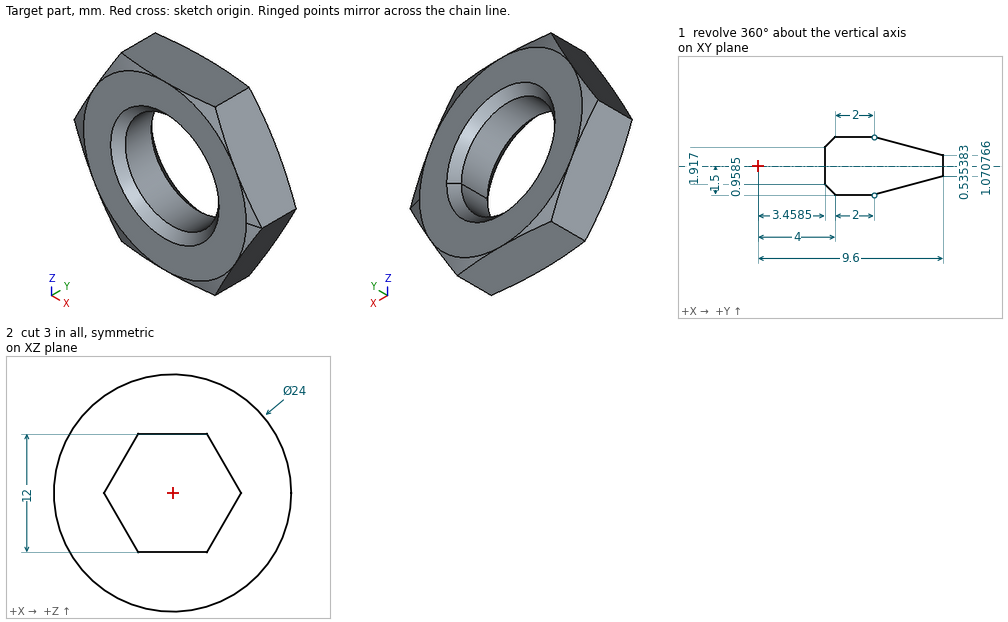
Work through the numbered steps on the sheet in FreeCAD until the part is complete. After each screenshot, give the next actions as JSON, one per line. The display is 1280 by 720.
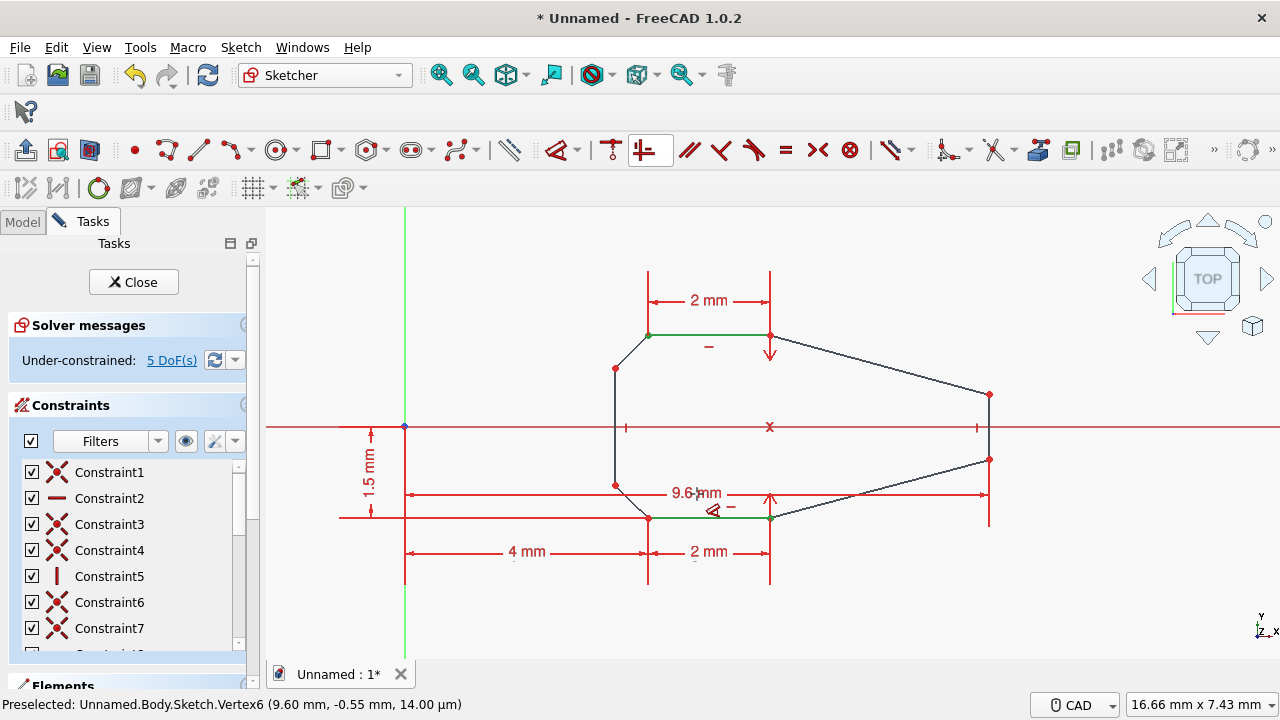
{"action": "left_click", "coordinate": [615, 404]}
{"action": "left_click", "coordinate": [581, 401]}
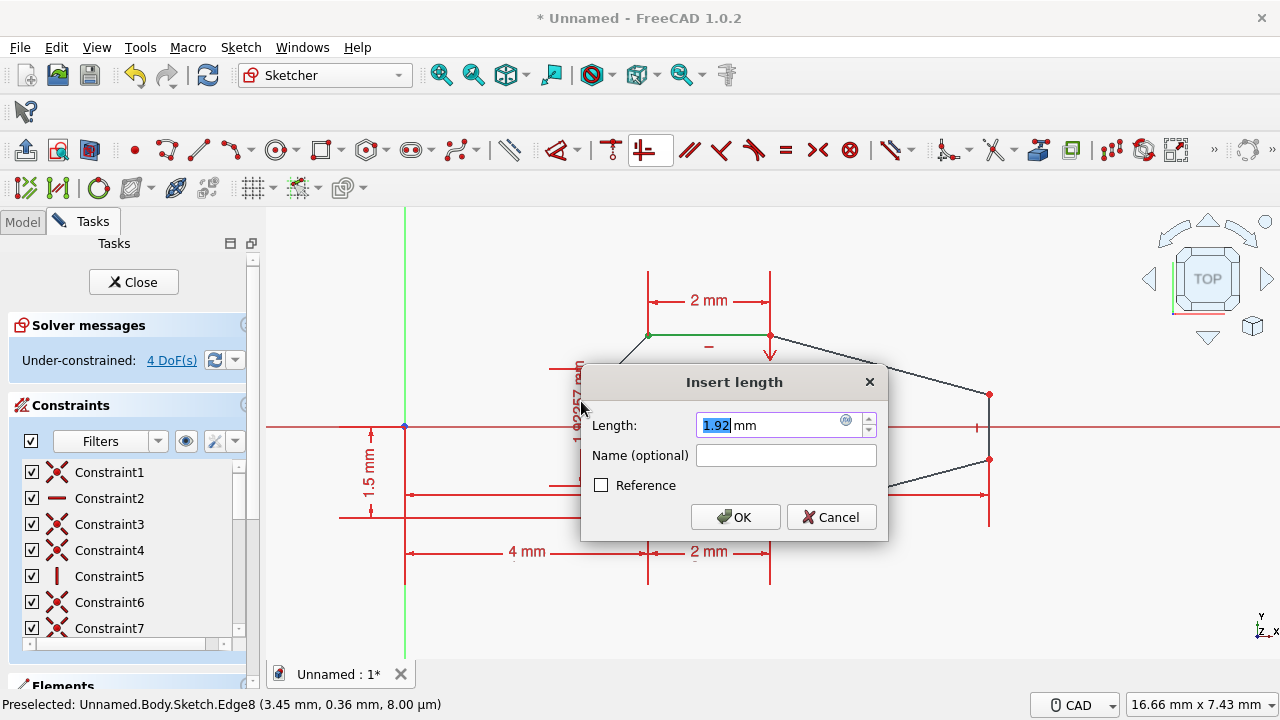
{"action": "type", "text": "1.917"}
{"action": "key", "text": "Return"}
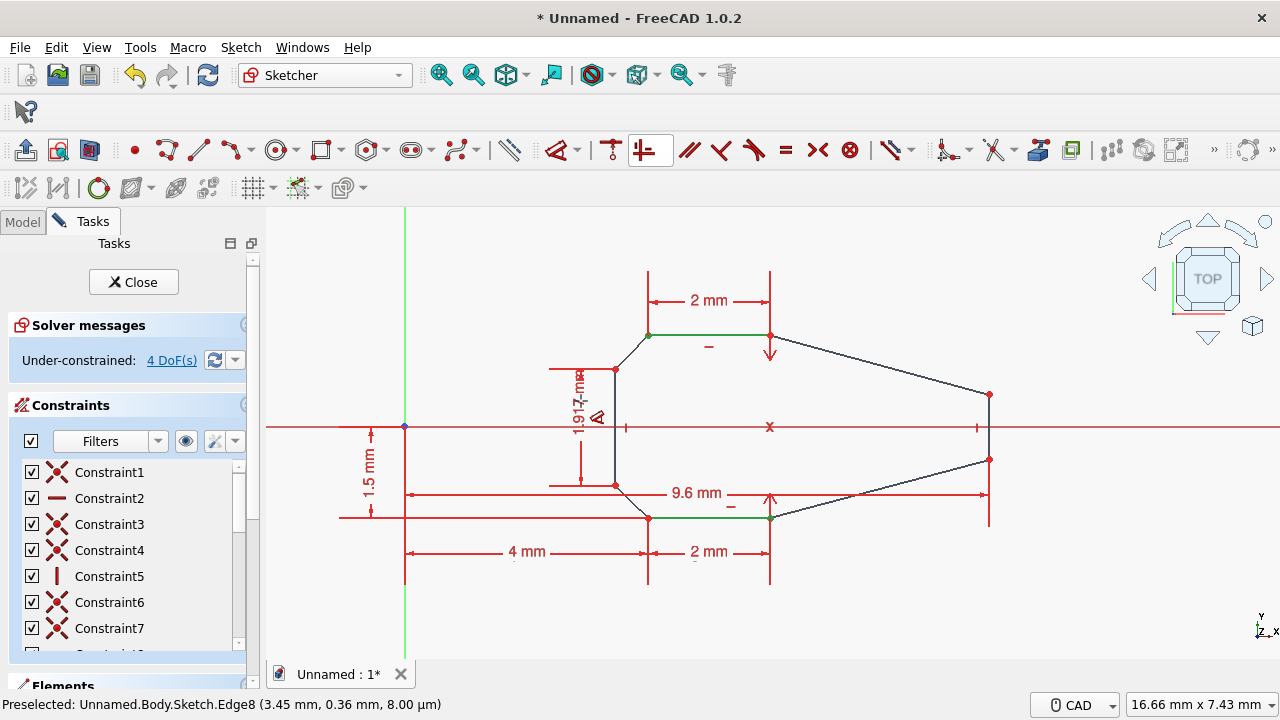
{"action": "left_click", "coordinate": [615, 486]}
{"action": "left_click", "coordinate": [510, 520]}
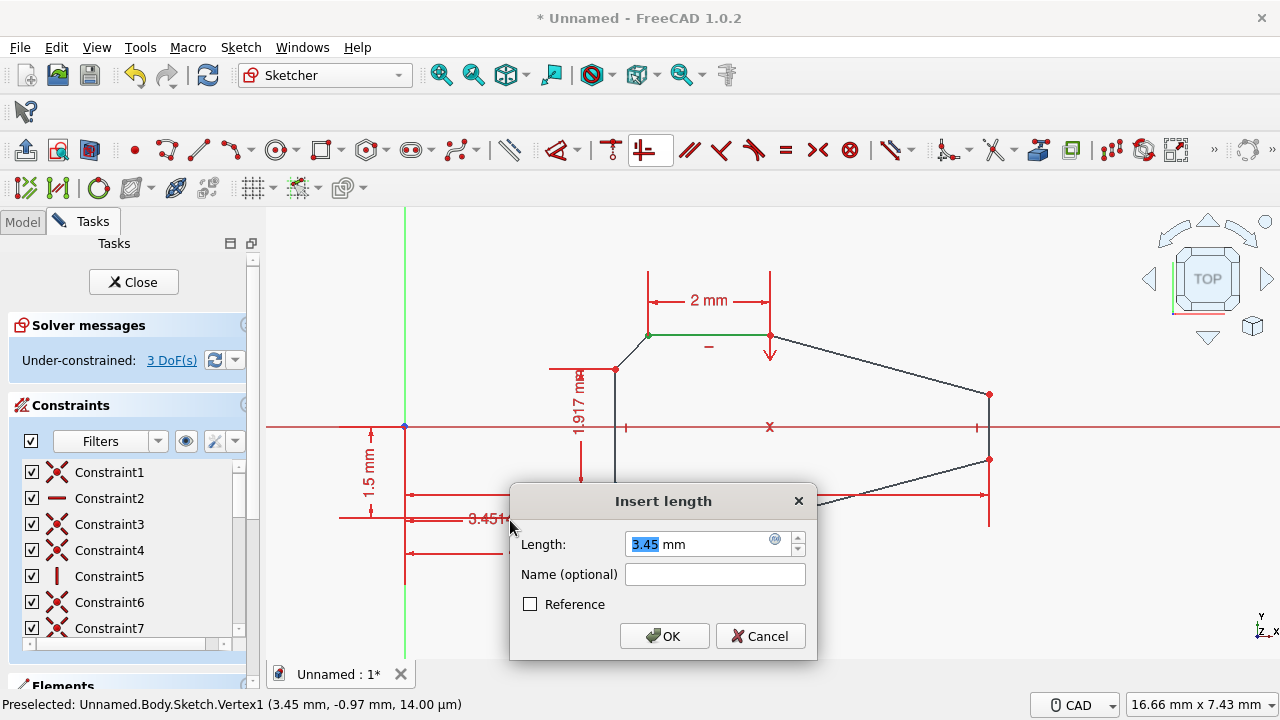
{"action": "type", "text": "3.4585"}
{"action": "key", "text": "Return"}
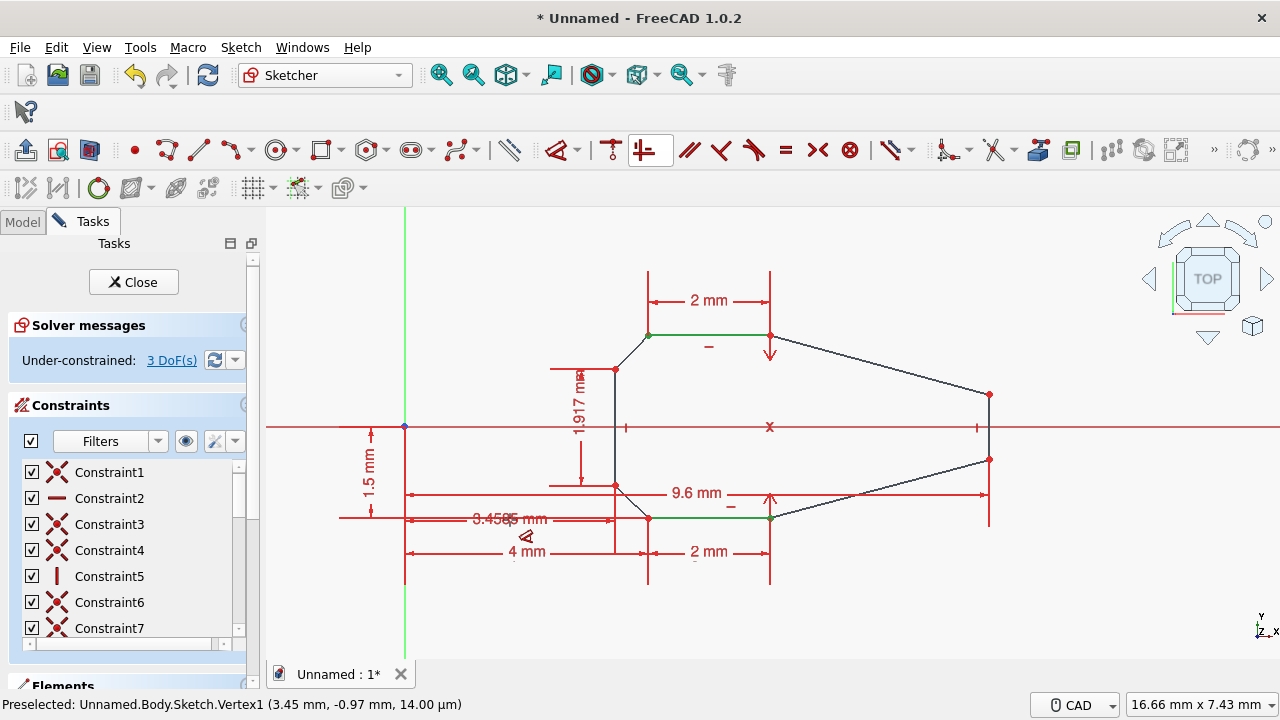
{"action": "left_click", "coordinate": [615, 486]}
{"action": "left_click", "coordinate": [371, 443]}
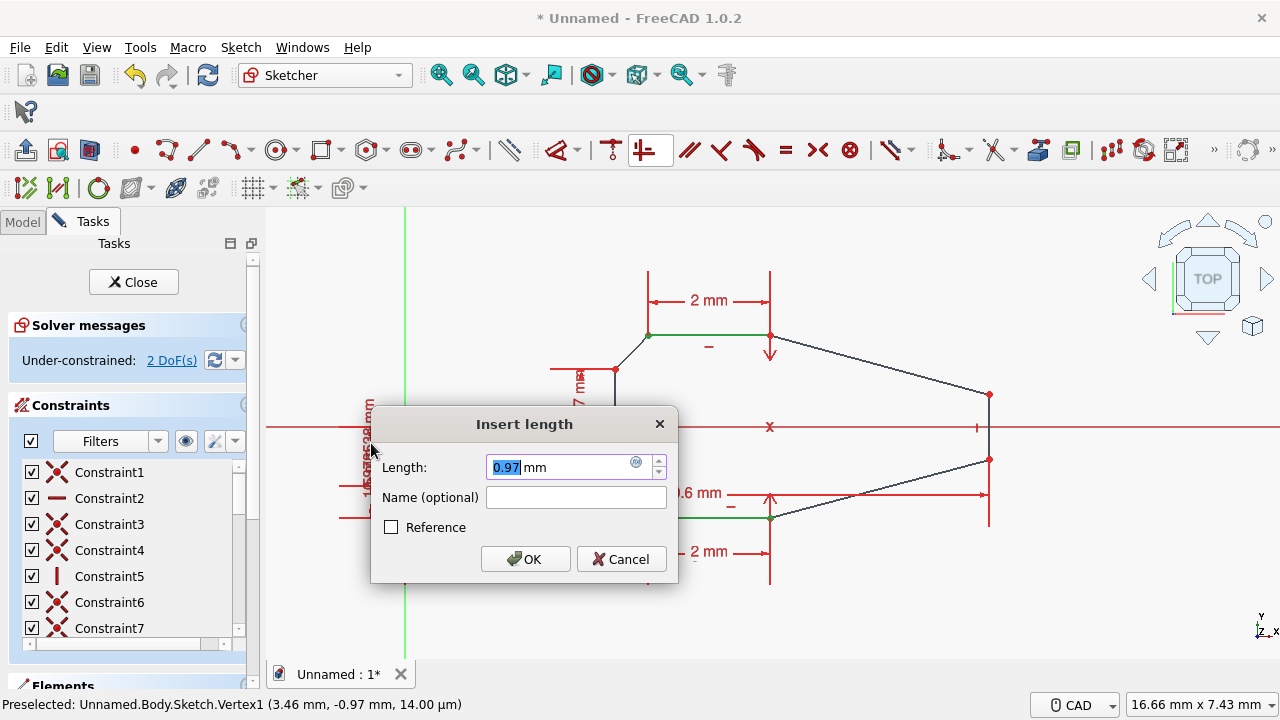
{"action": "type", "text": "0.9585"}
{"action": "key", "text": "Return"}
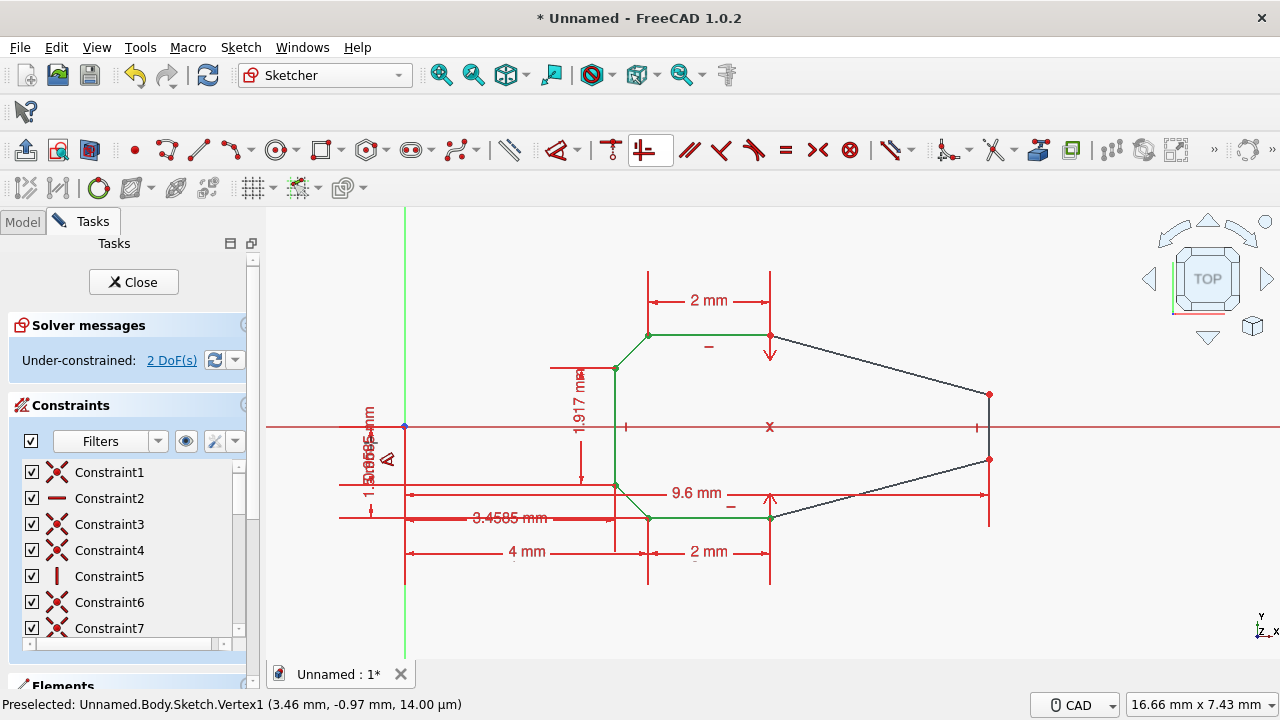
{"action": "left_click", "coordinate": [989, 440]}
{"action": "left_click", "coordinate": [1023, 413]}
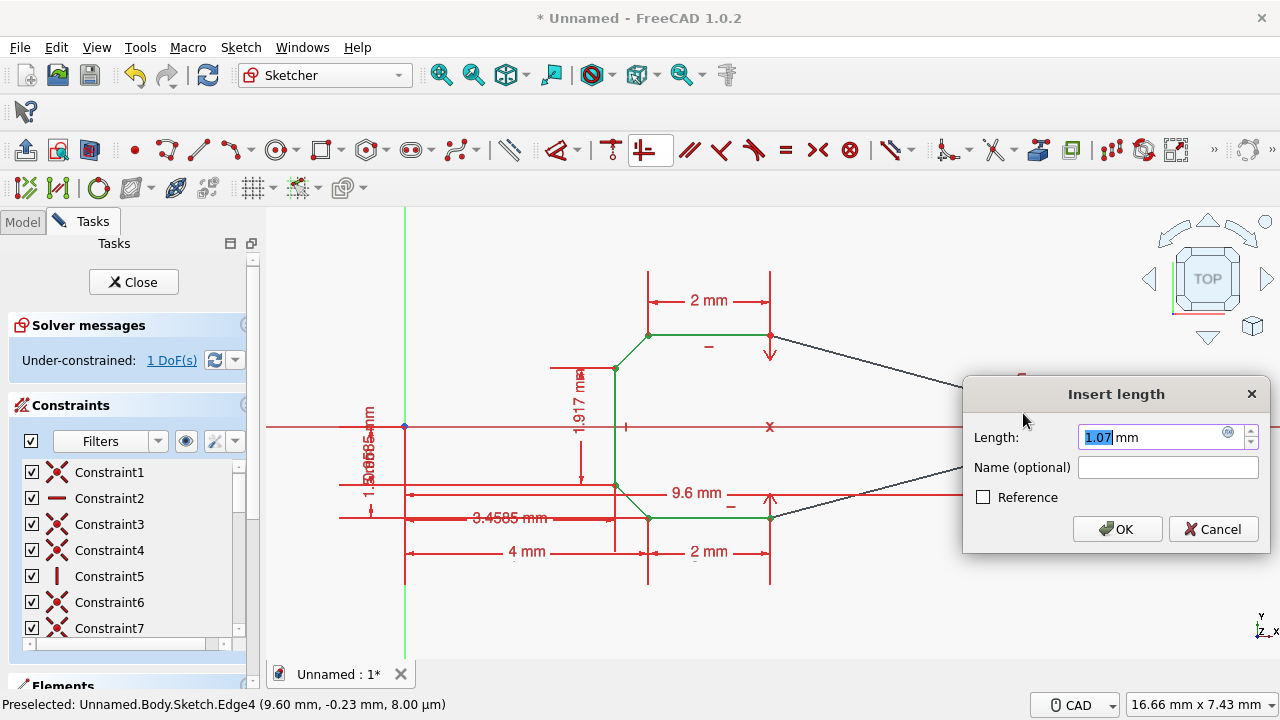
{"action": "type", "text": "1.070766"}
{"action": "key", "text": "Return"}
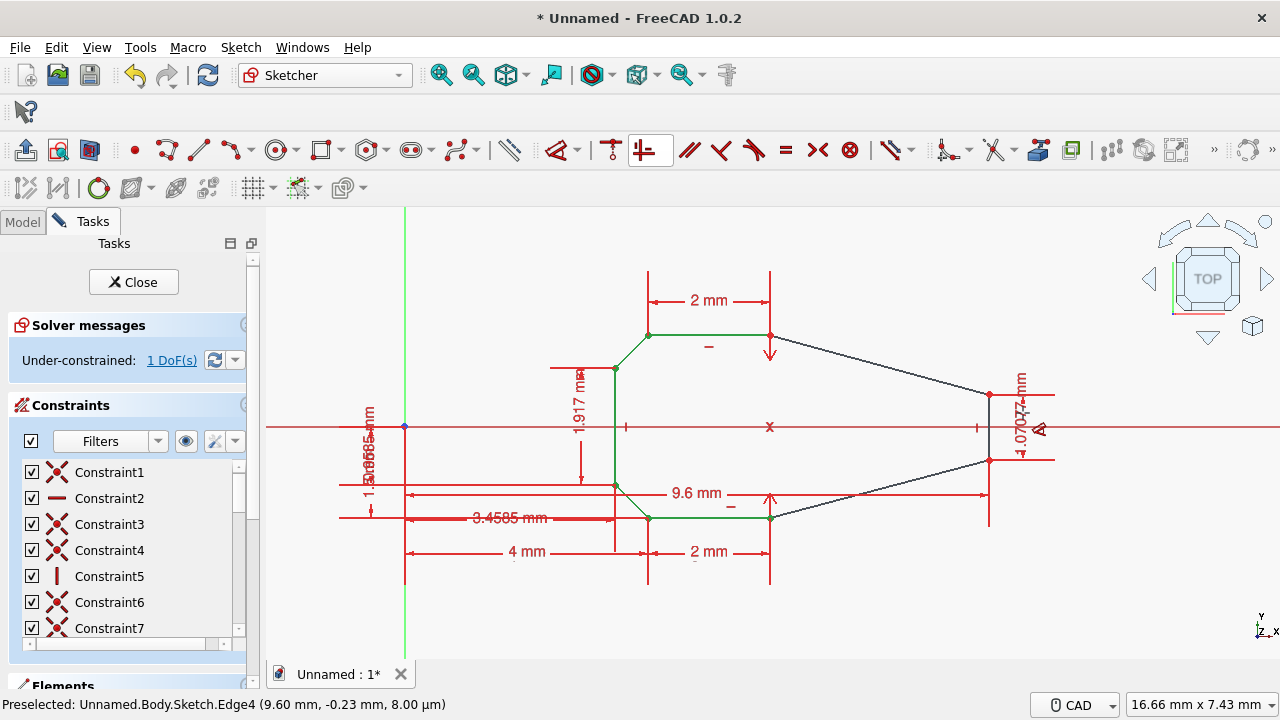
{"action": "left_click", "coordinate": [989, 460]}
{"action": "left_click", "coordinate": [1023, 443]}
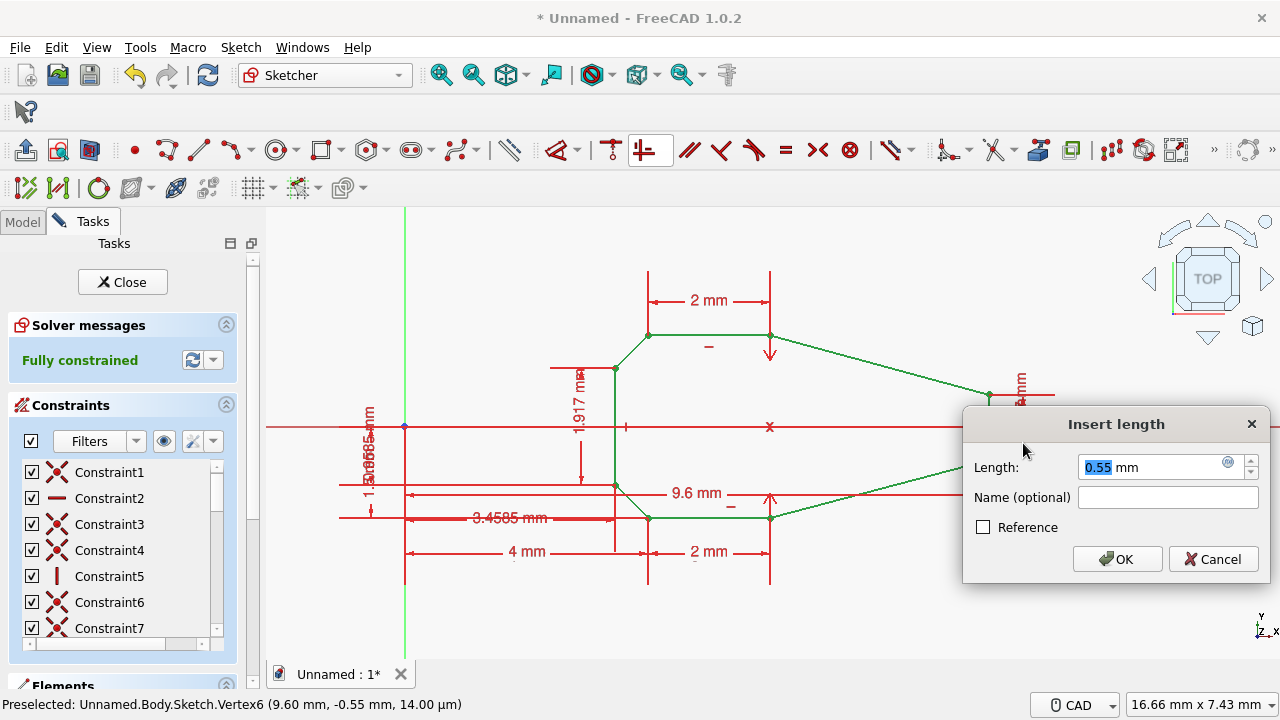
{"action": "type", "text": "0.535383"}
{"action": "key", "text": "Return"}
{"action": "key", "text": "Escape"}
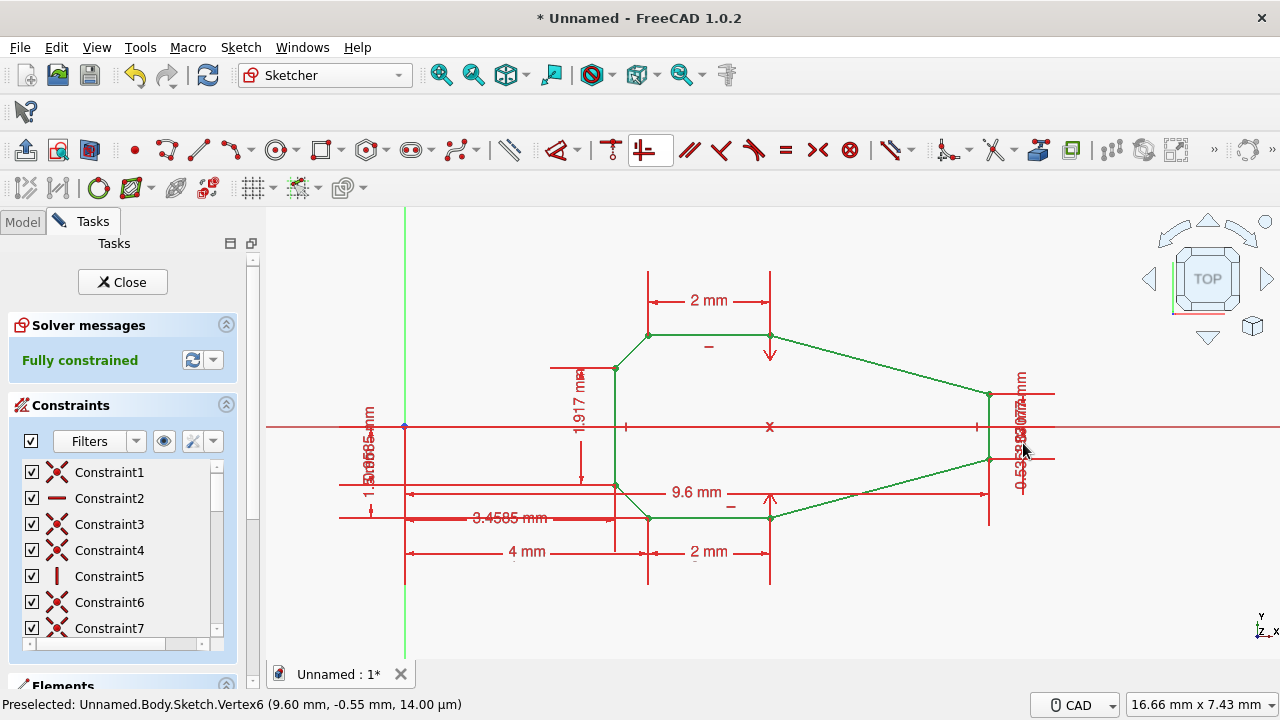
{"action": "left_click", "coordinate": [123, 282]}